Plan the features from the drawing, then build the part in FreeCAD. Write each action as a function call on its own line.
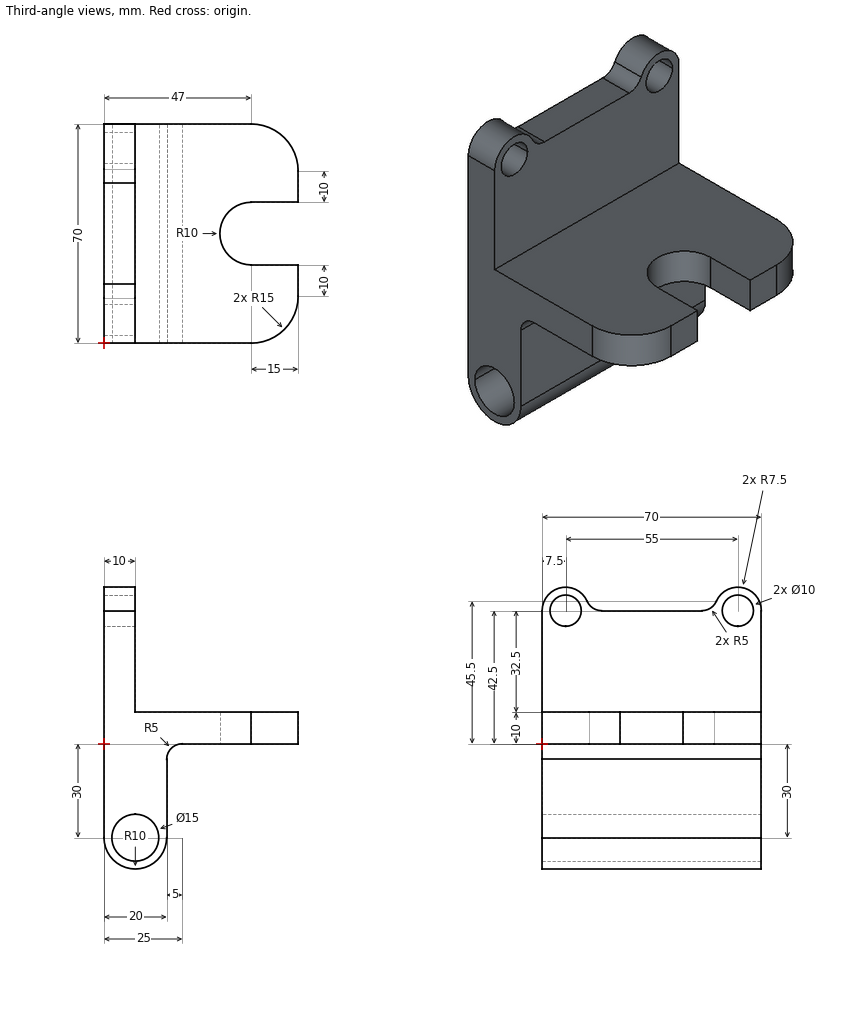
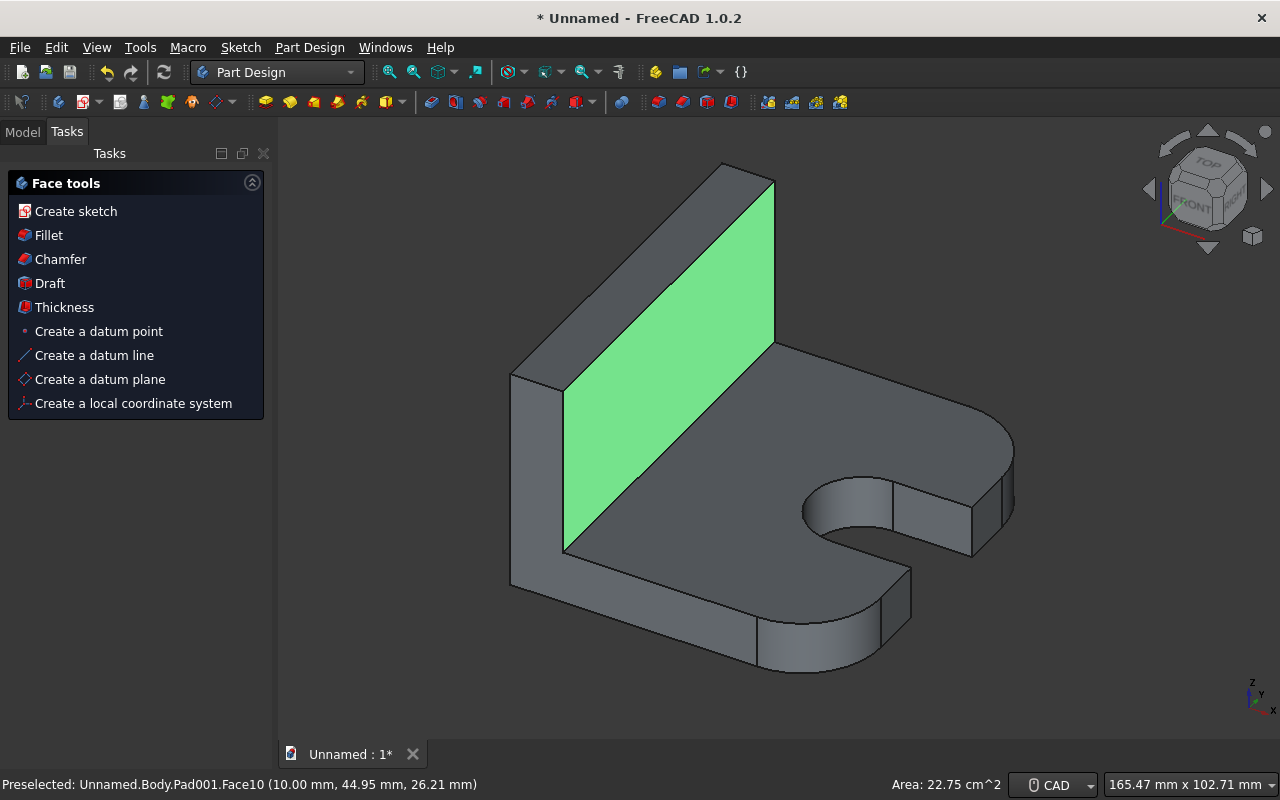
click(84, 102)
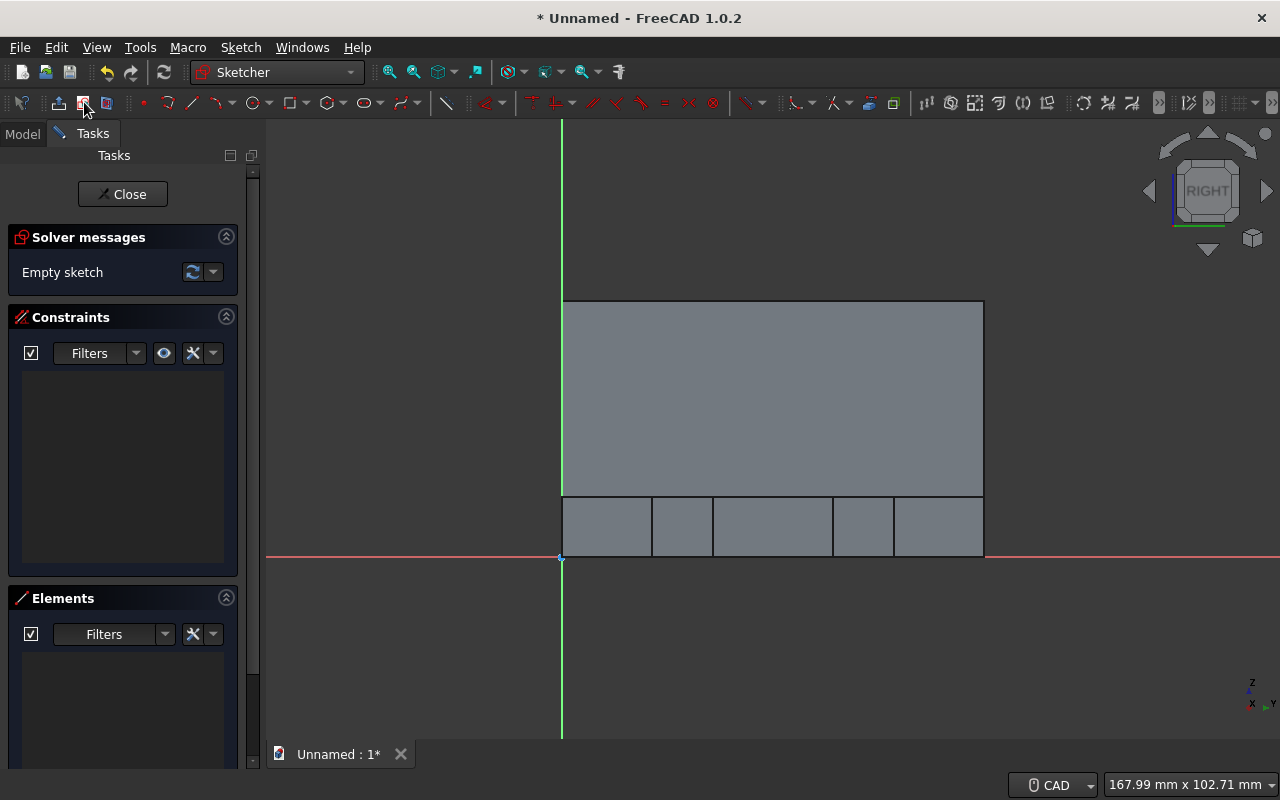
click(108, 104)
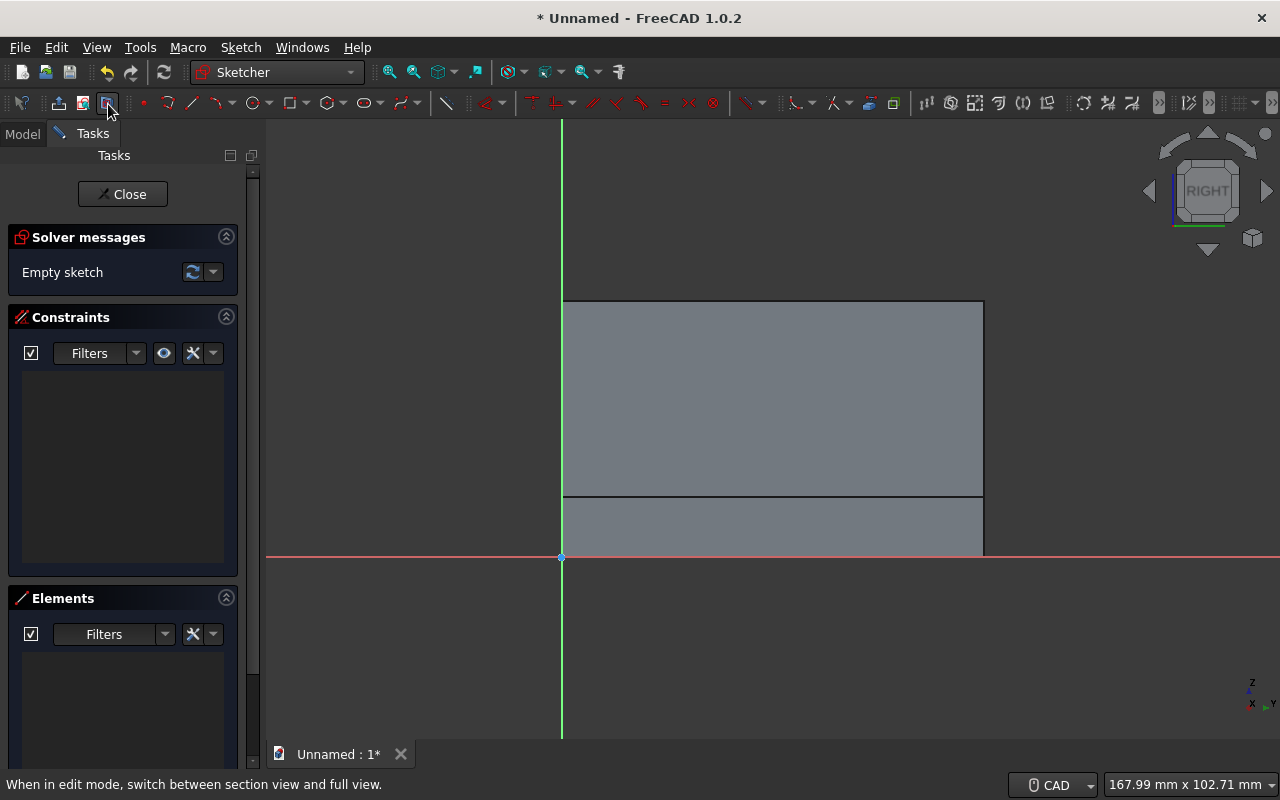
click(192, 104)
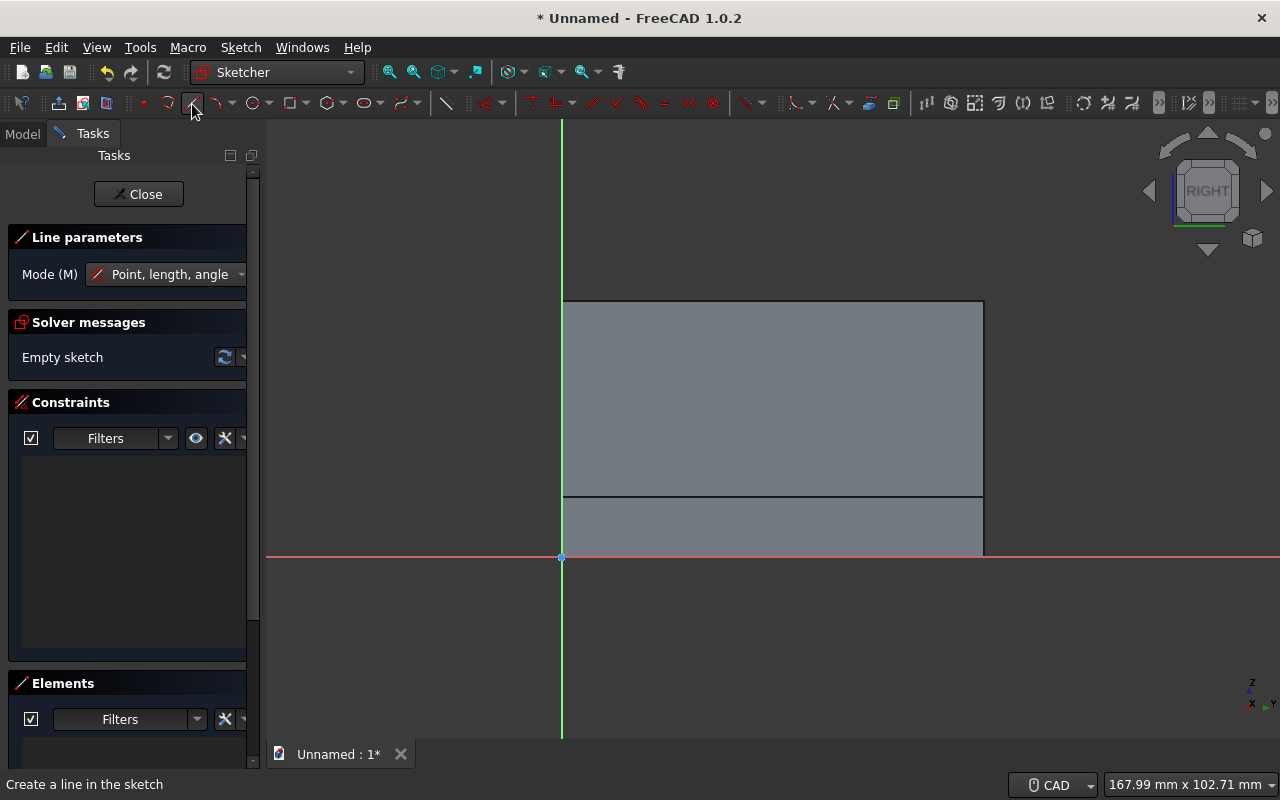
click(870, 301)
click(984, 301)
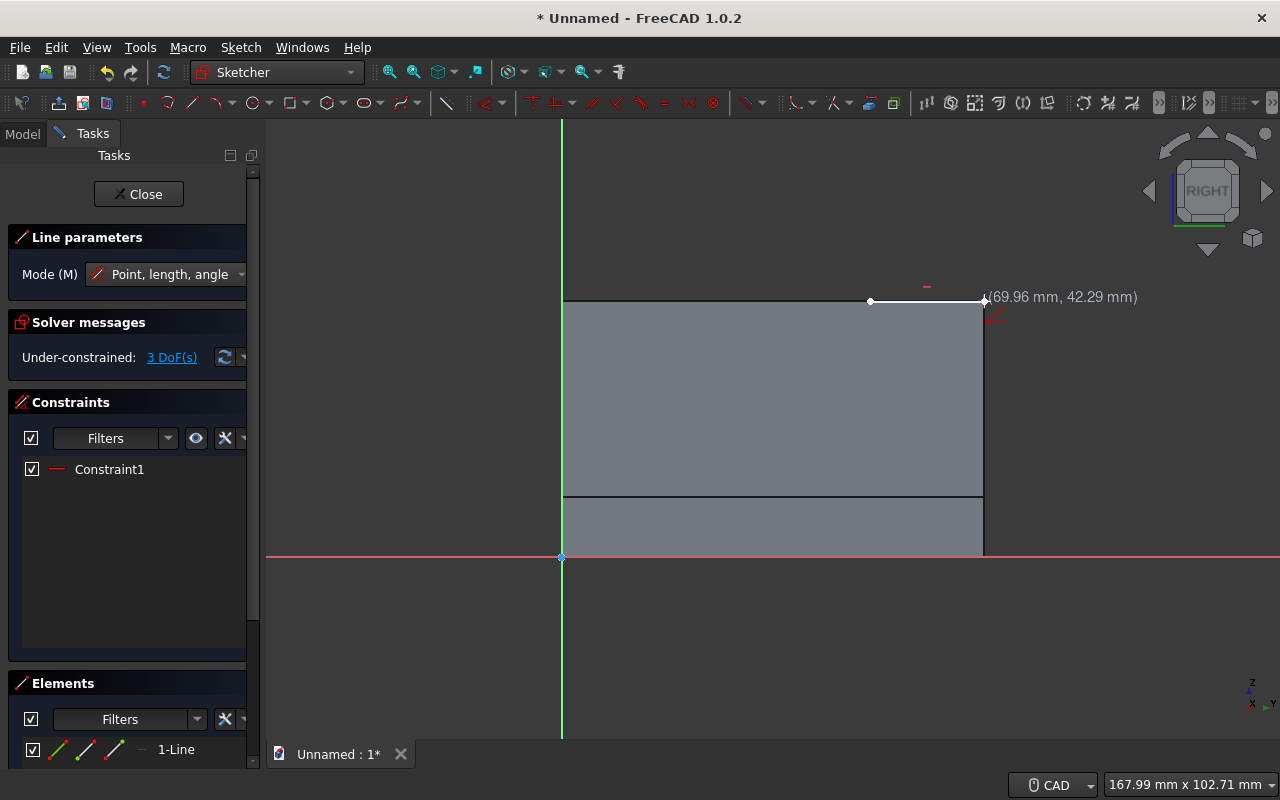
click(216, 104)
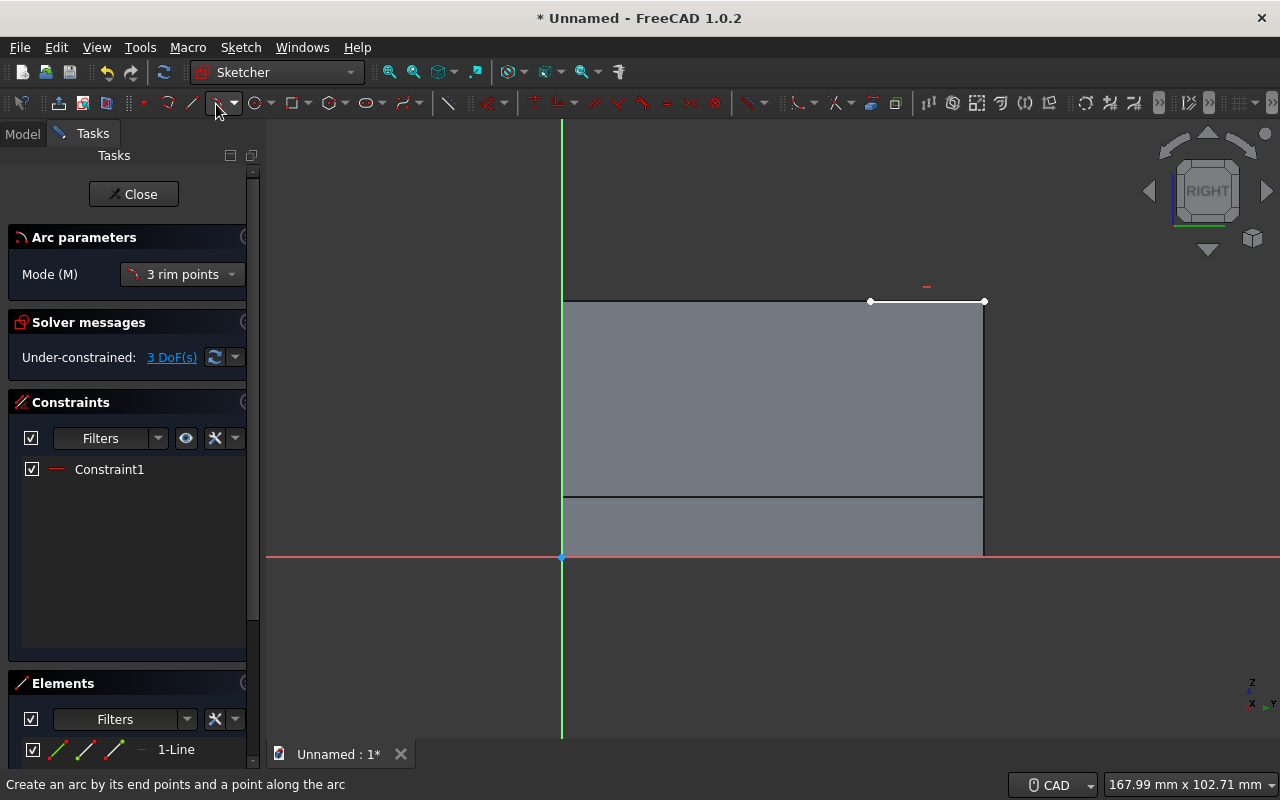
click(984, 302)
click(898, 283)
click(948, 256)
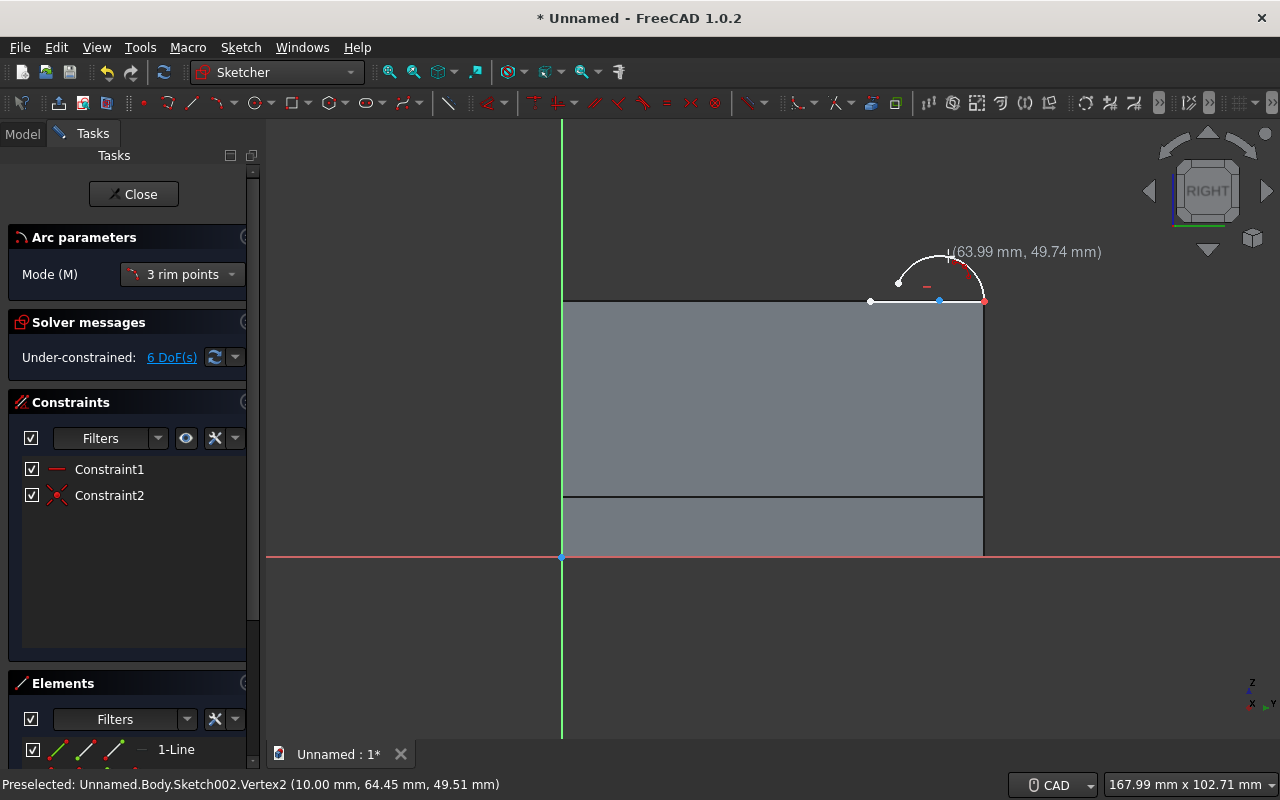
click(898, 284)
click(870, 302)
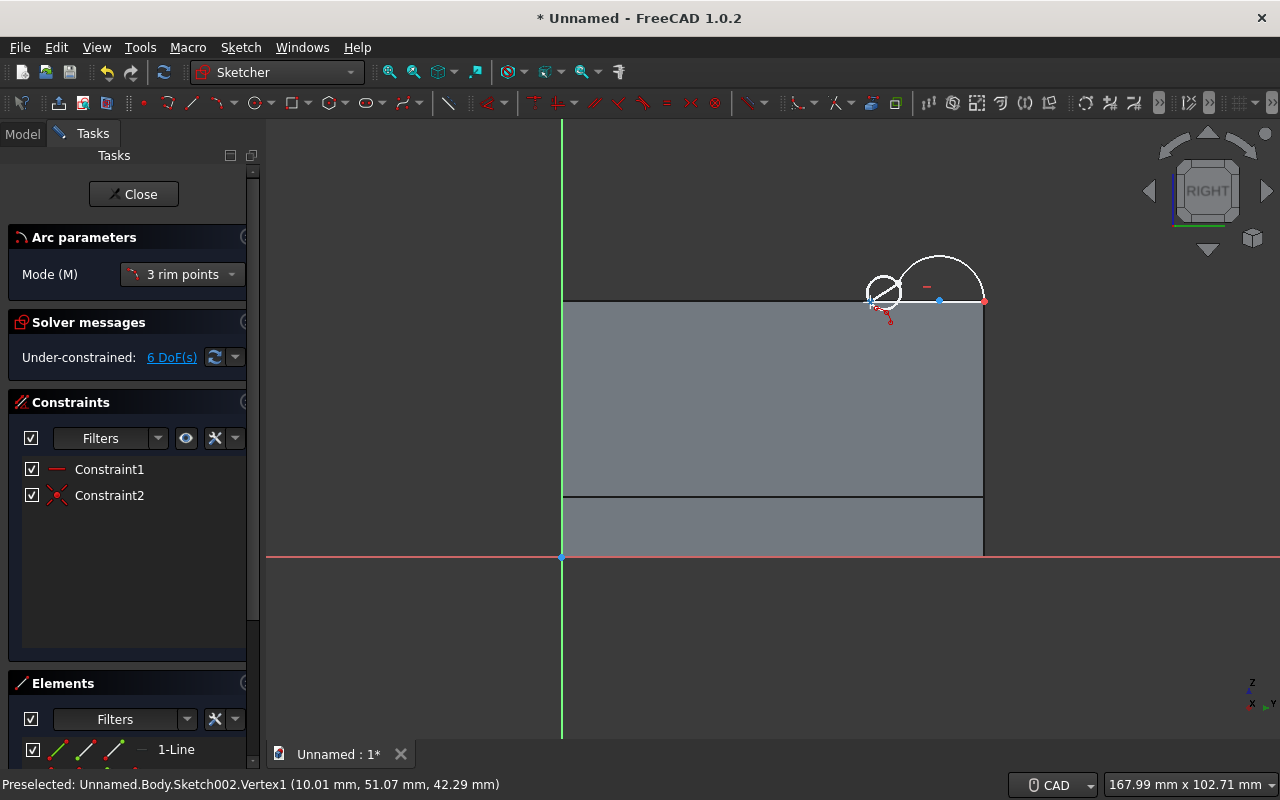
scroll(886, 296, up, 6)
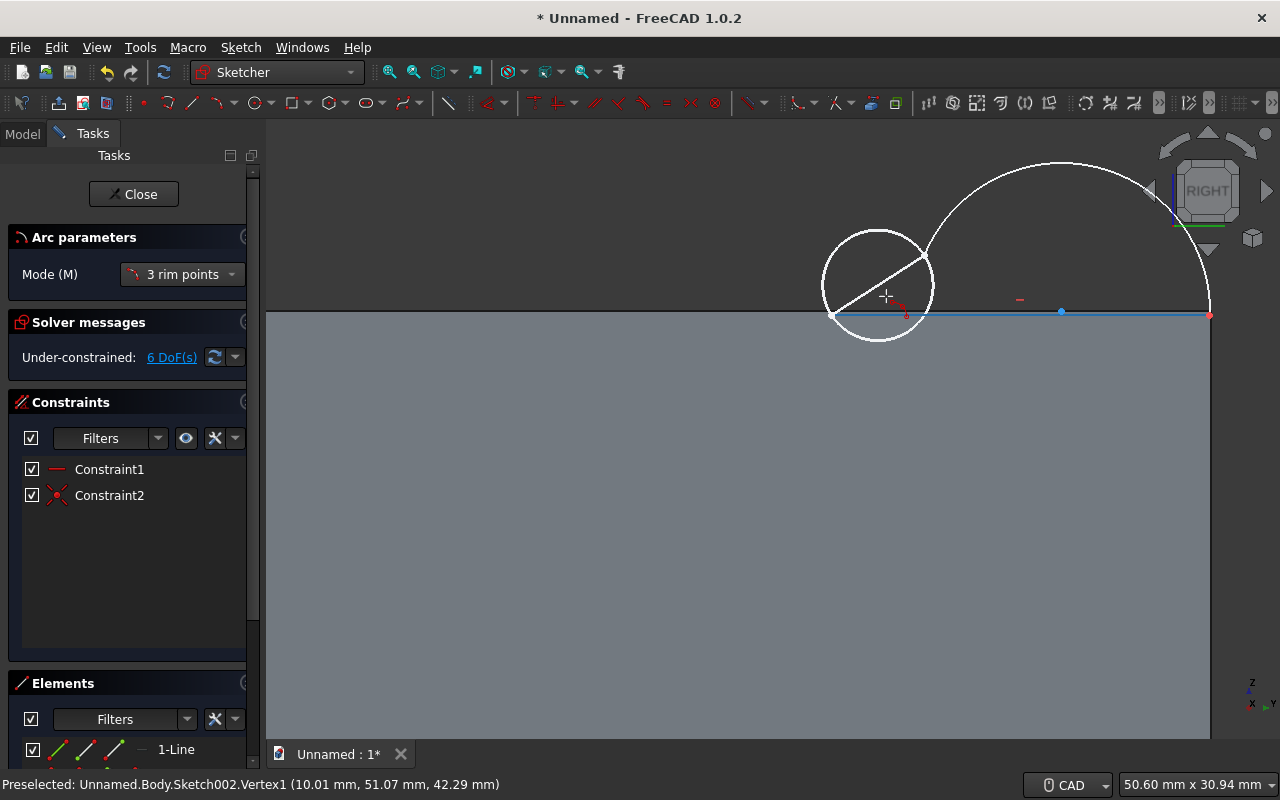
click(886, 295)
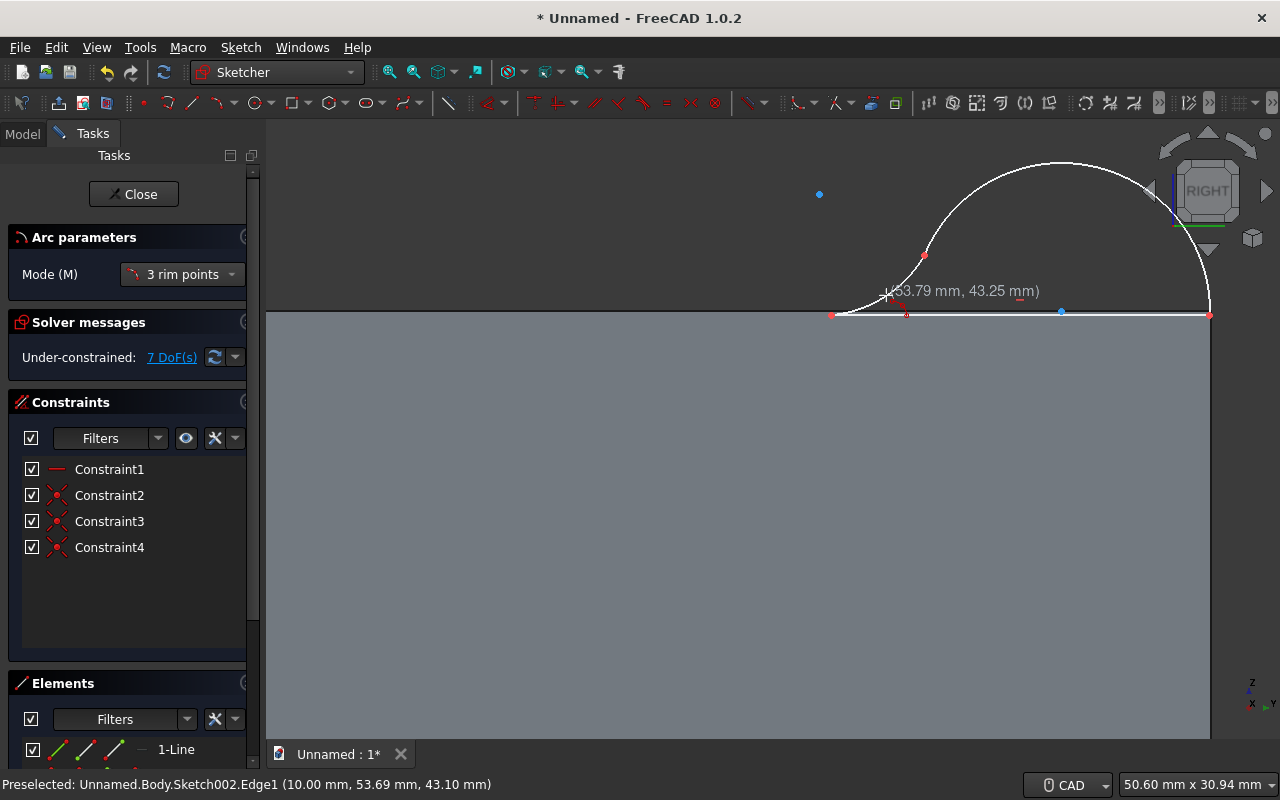
click(192, 104)